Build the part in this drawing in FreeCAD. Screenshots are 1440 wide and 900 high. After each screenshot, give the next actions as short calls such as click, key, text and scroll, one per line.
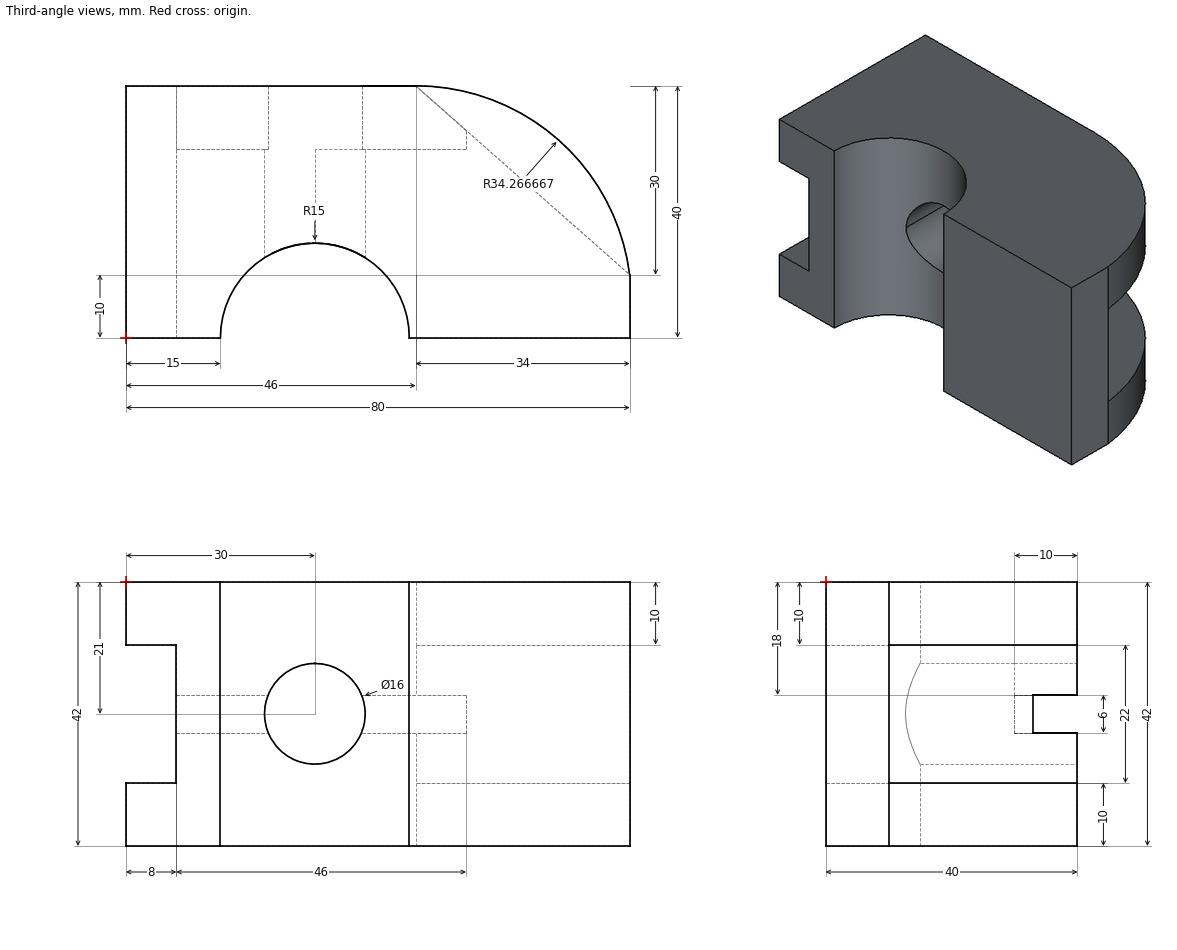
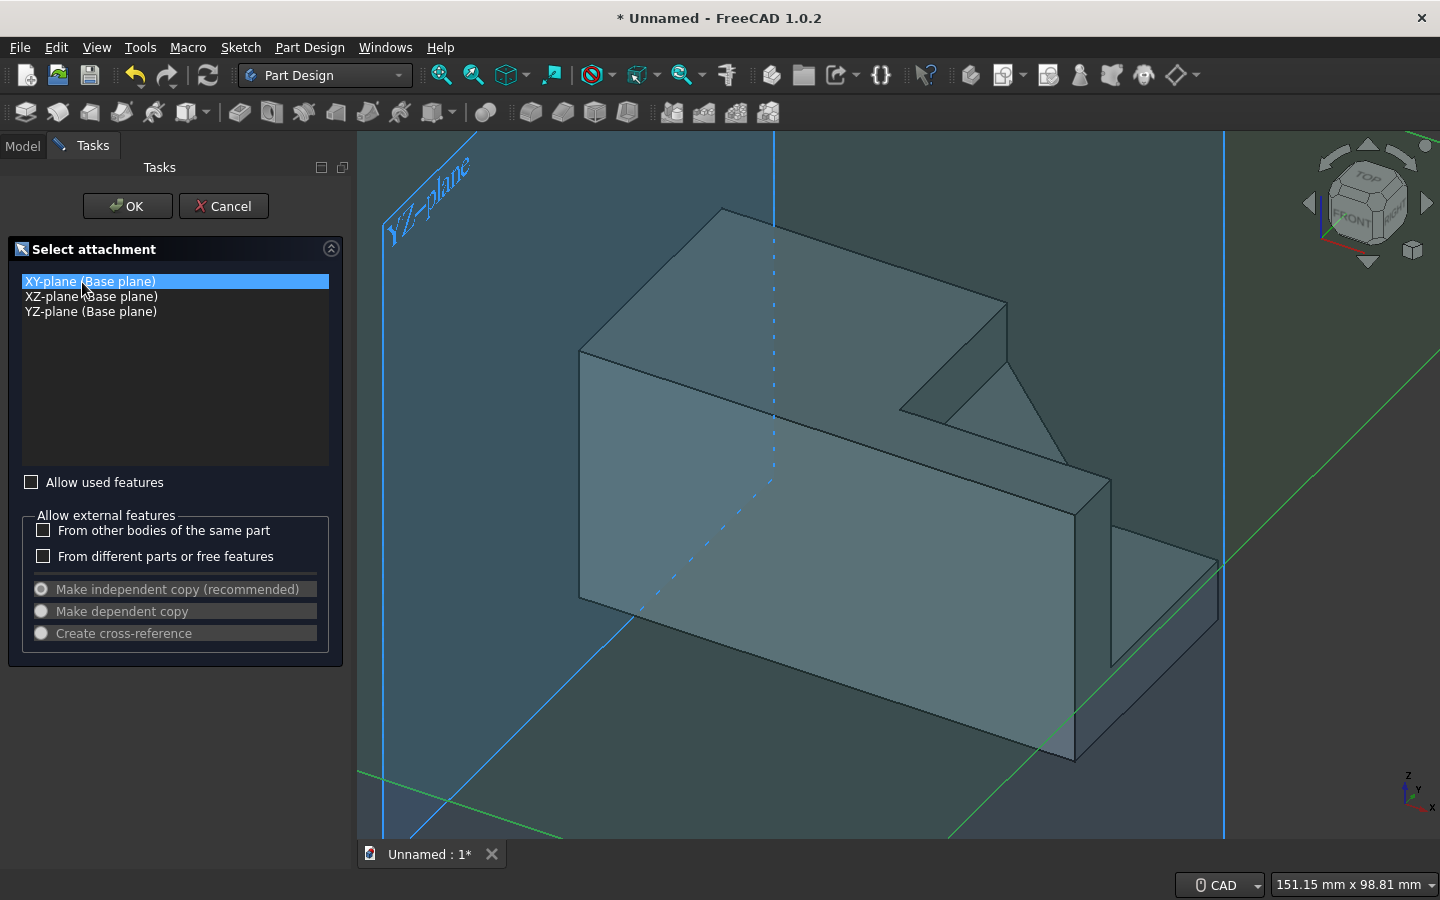
click(128, 206)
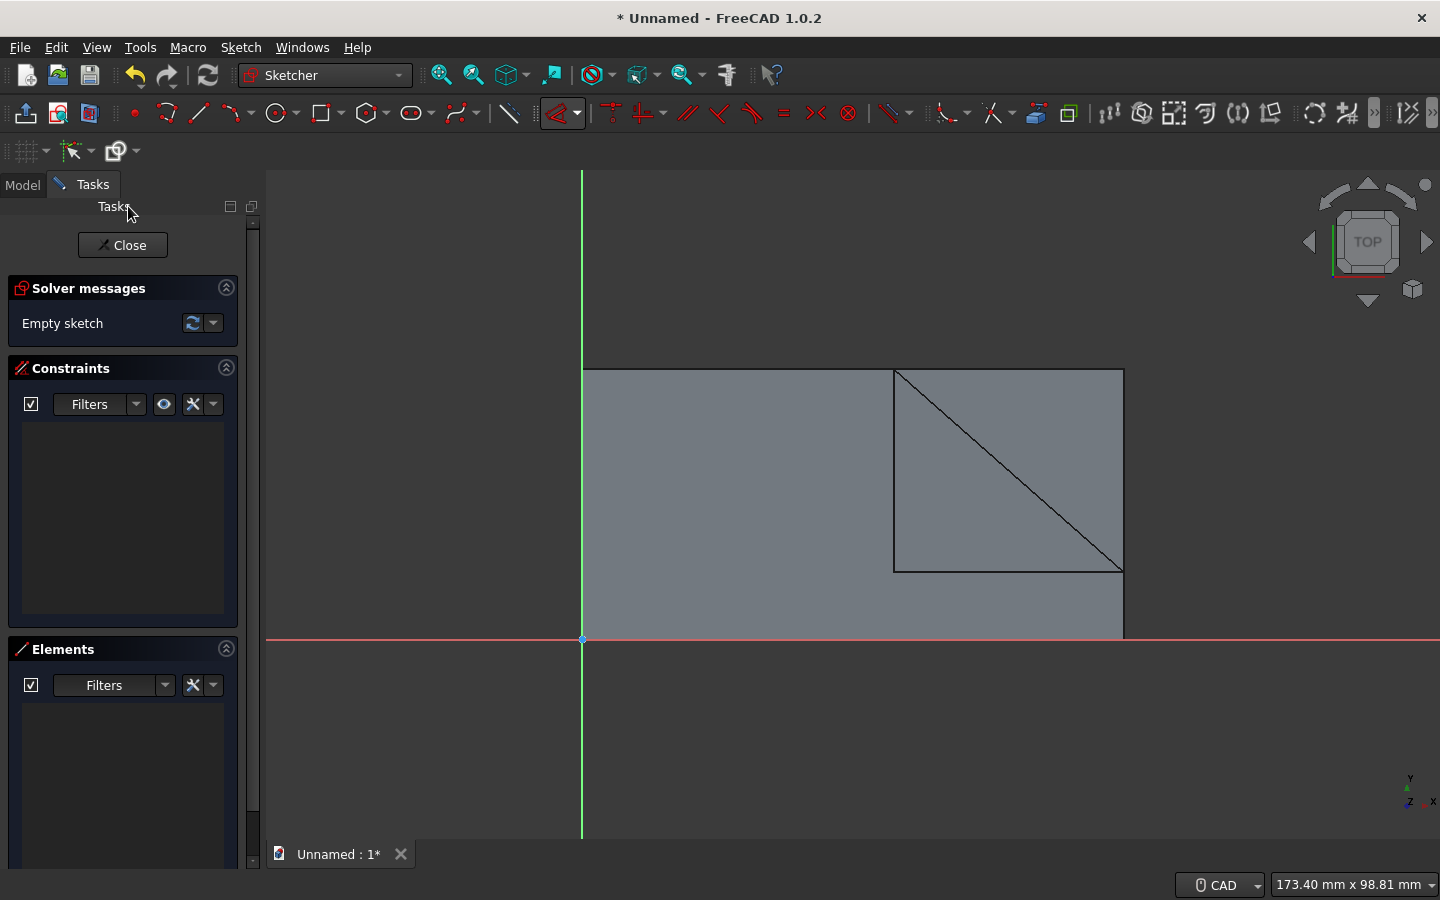
click(168, 114)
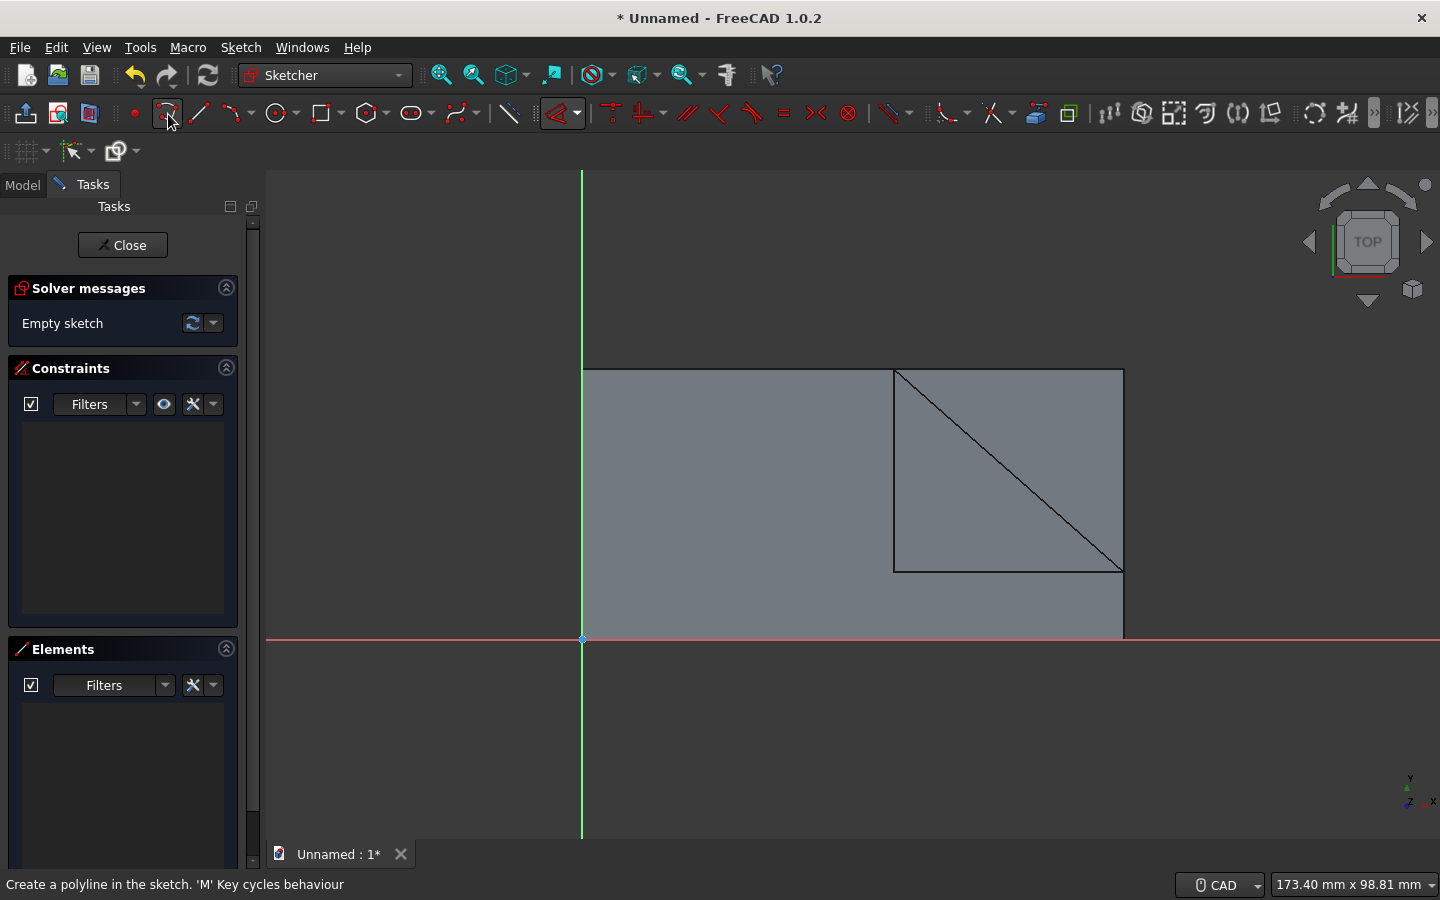
click(894, 369)
click(894, 572)
click(1124, 572)
right_click(1124, 572)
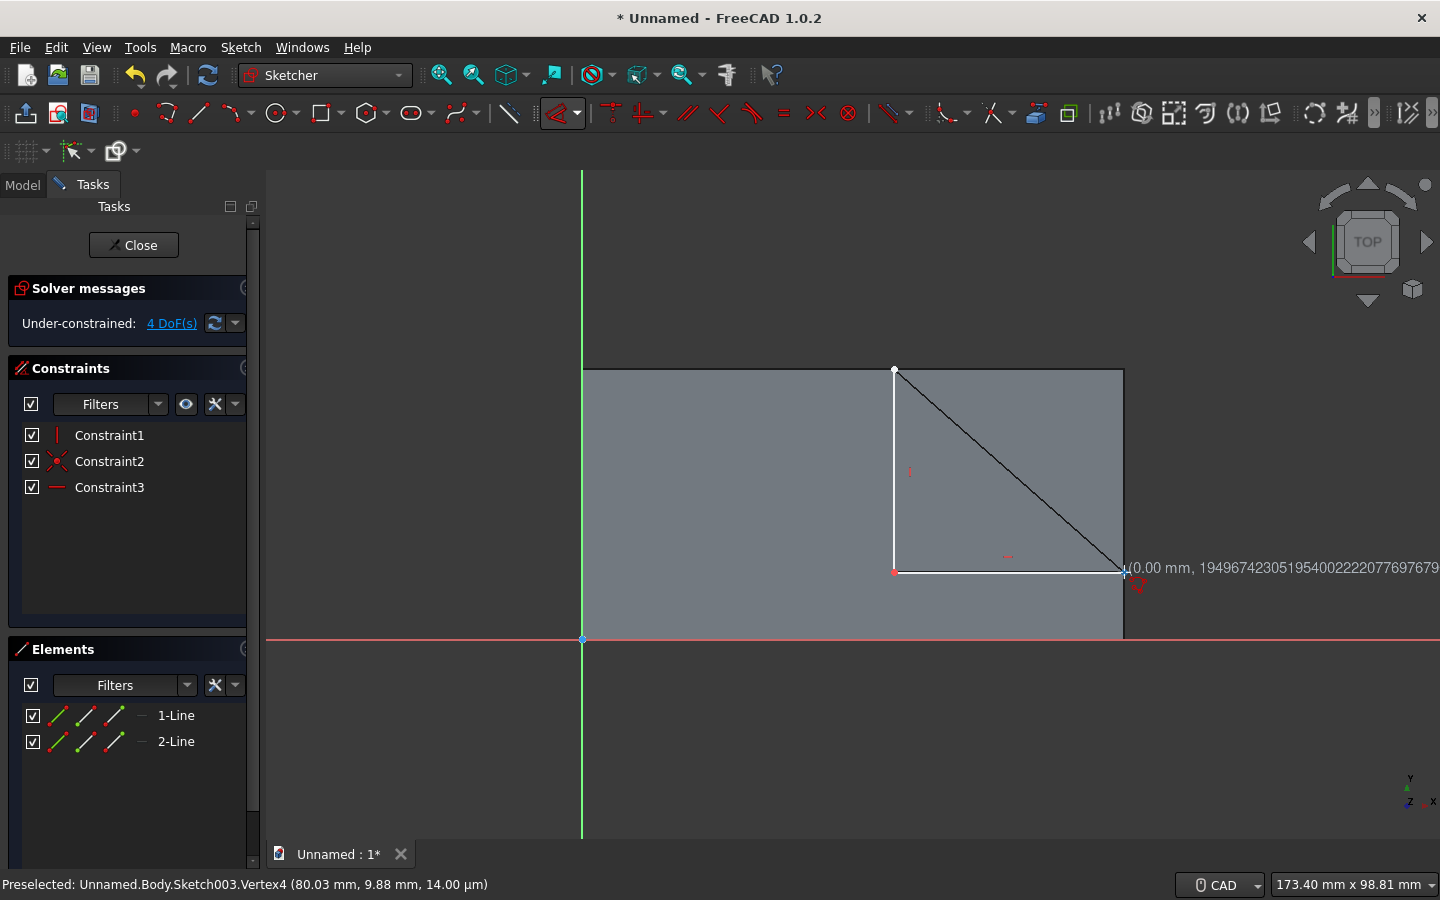
click(232, 114)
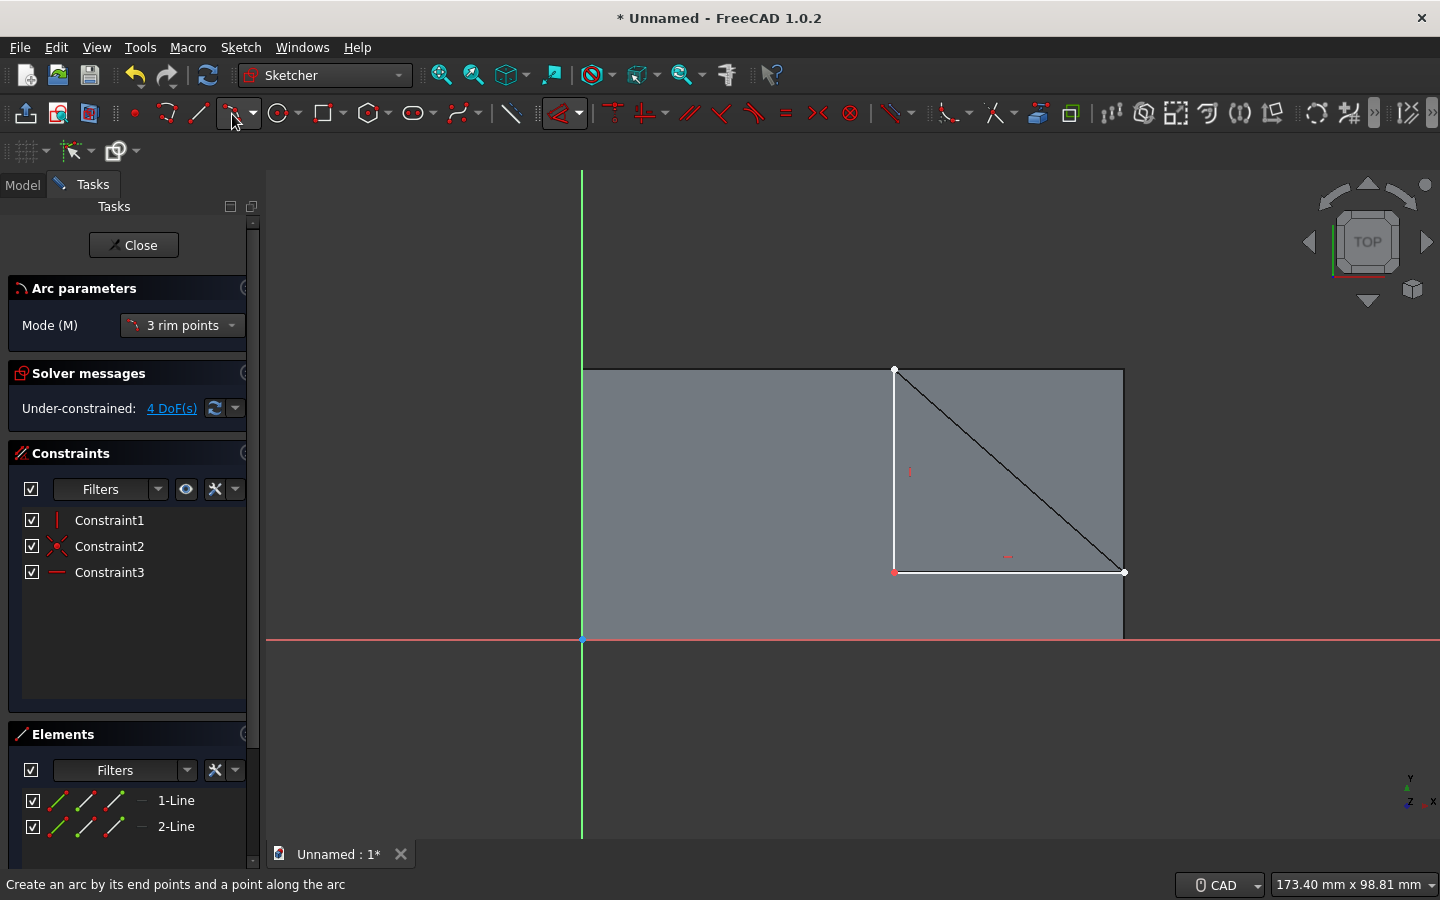
click(1124, 573)
click(894, 370)
click(1047, 427)
key(Escape)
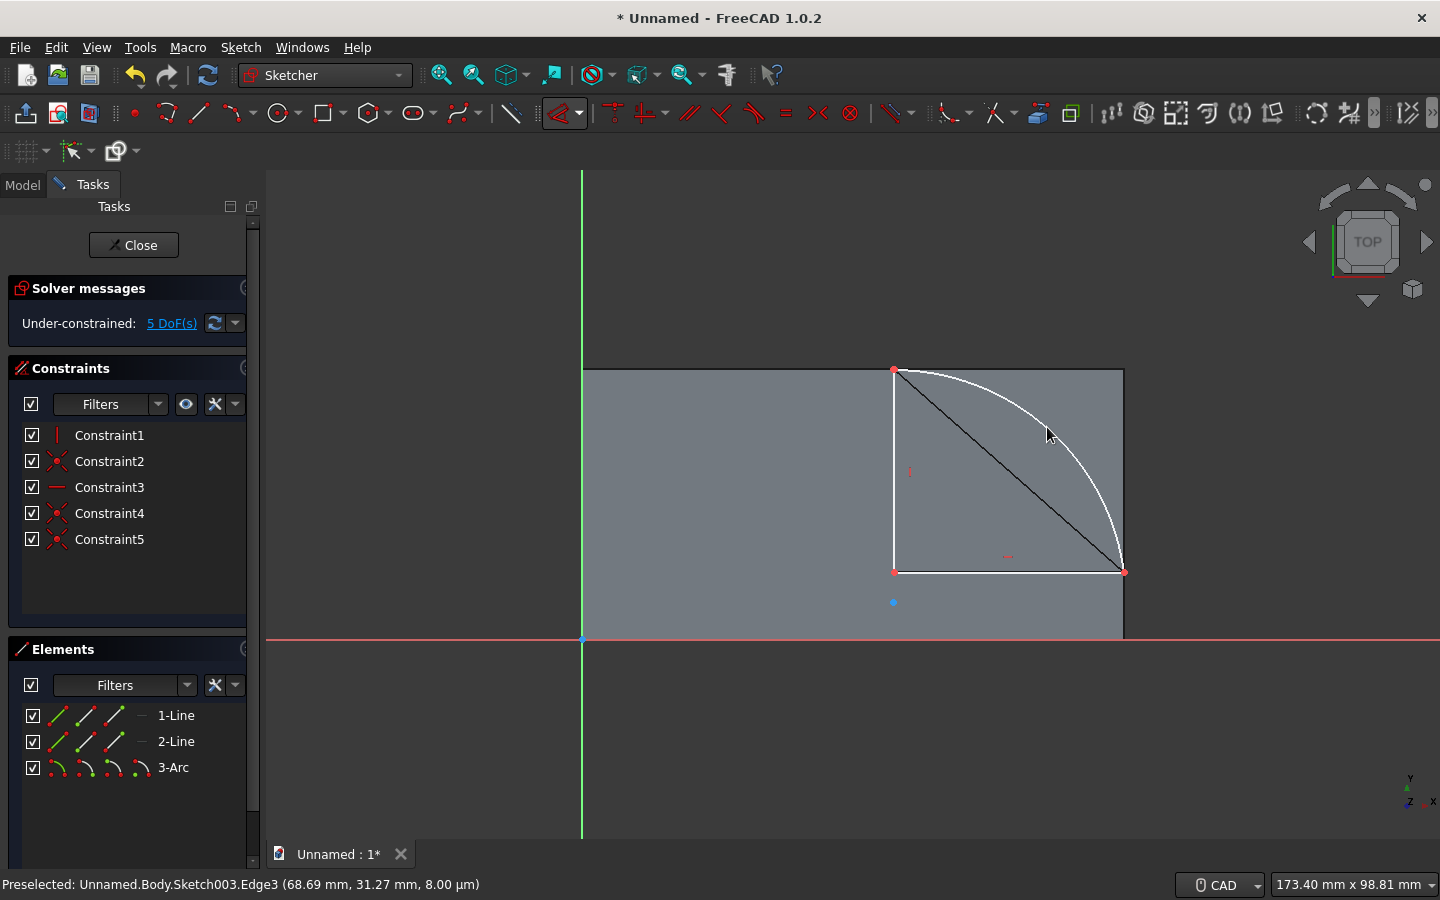
click(1090, 479)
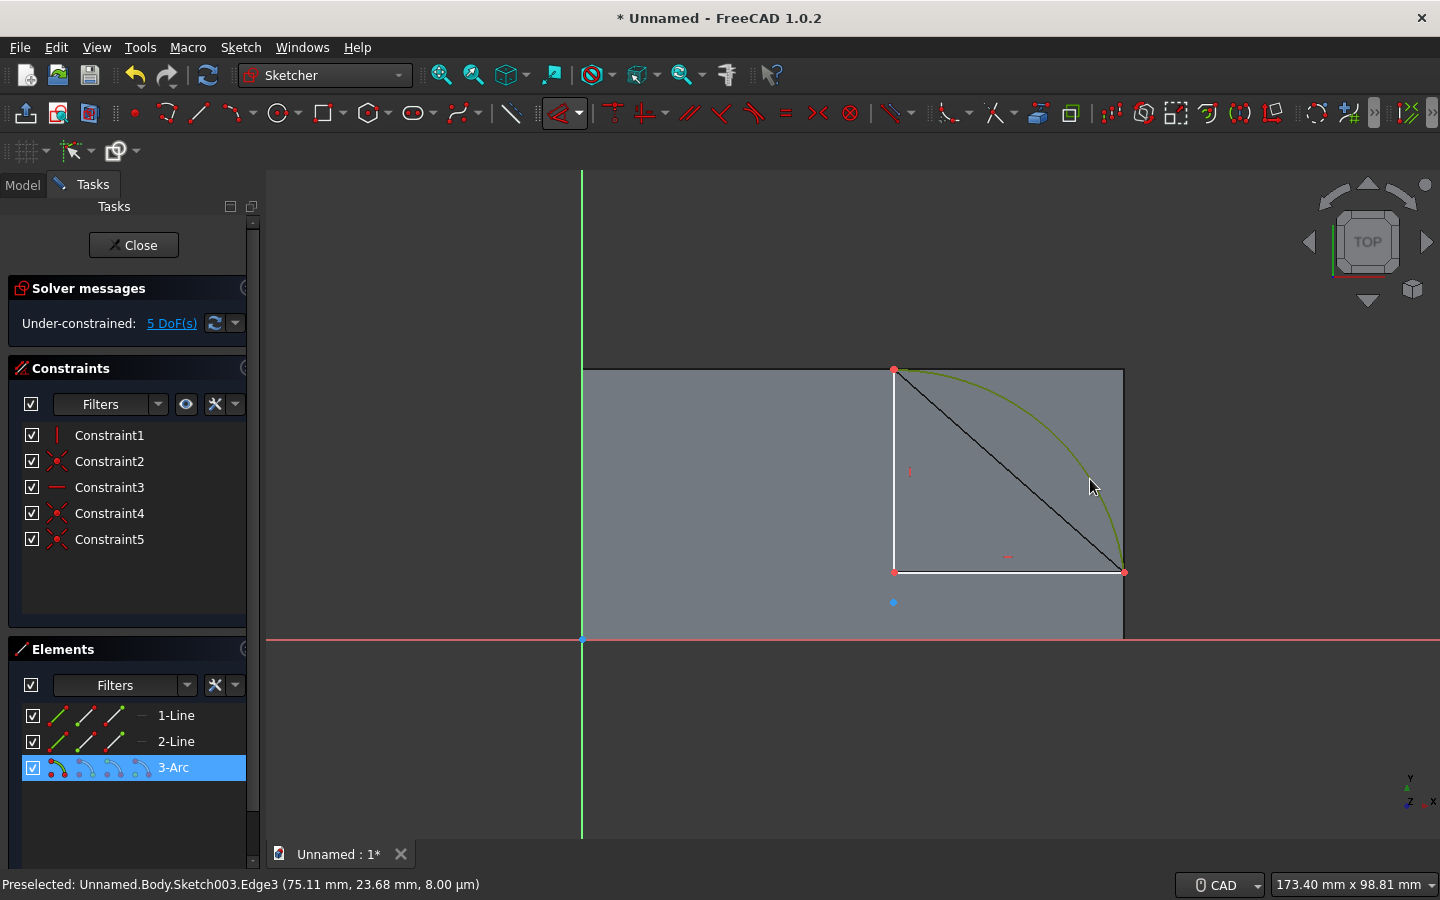
click(582, 114)